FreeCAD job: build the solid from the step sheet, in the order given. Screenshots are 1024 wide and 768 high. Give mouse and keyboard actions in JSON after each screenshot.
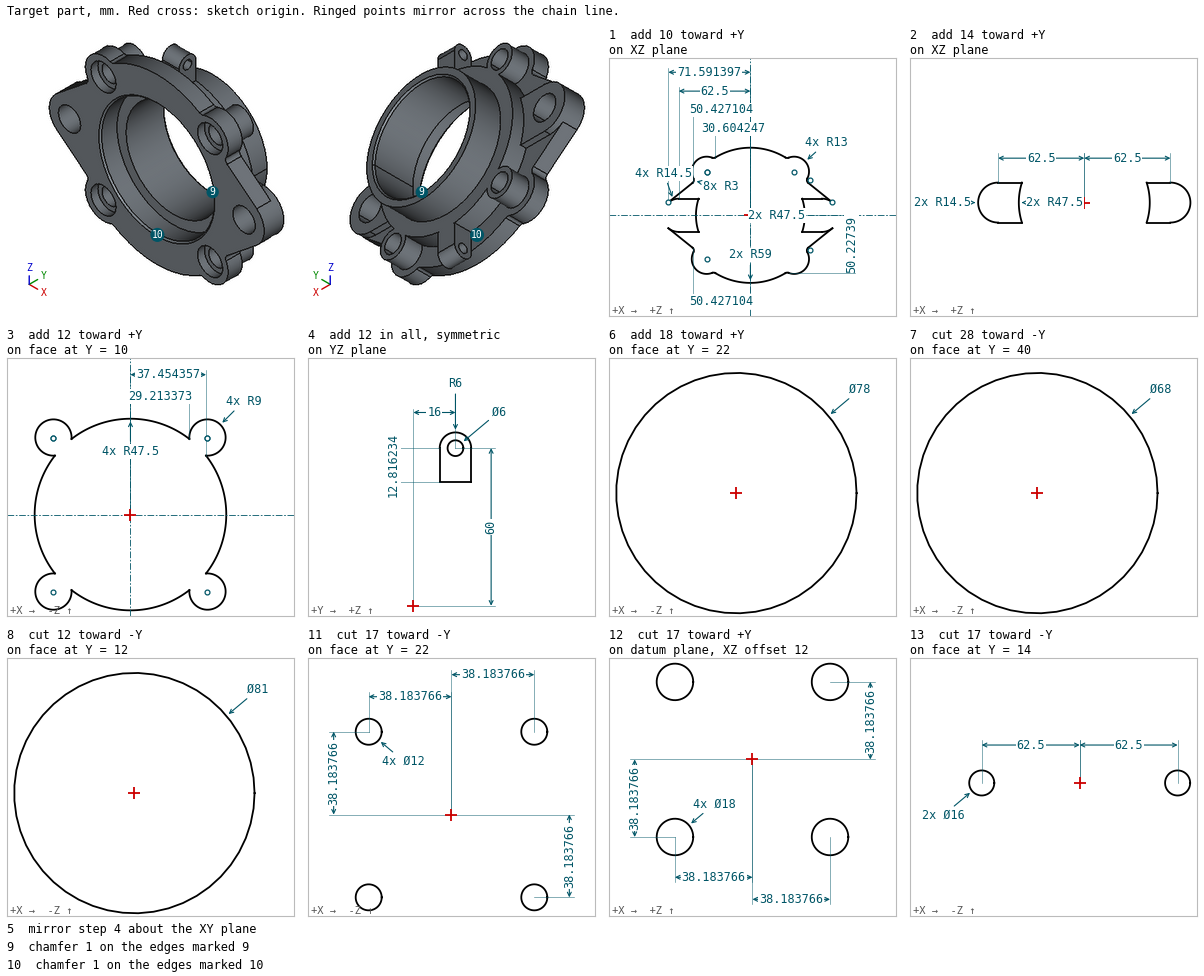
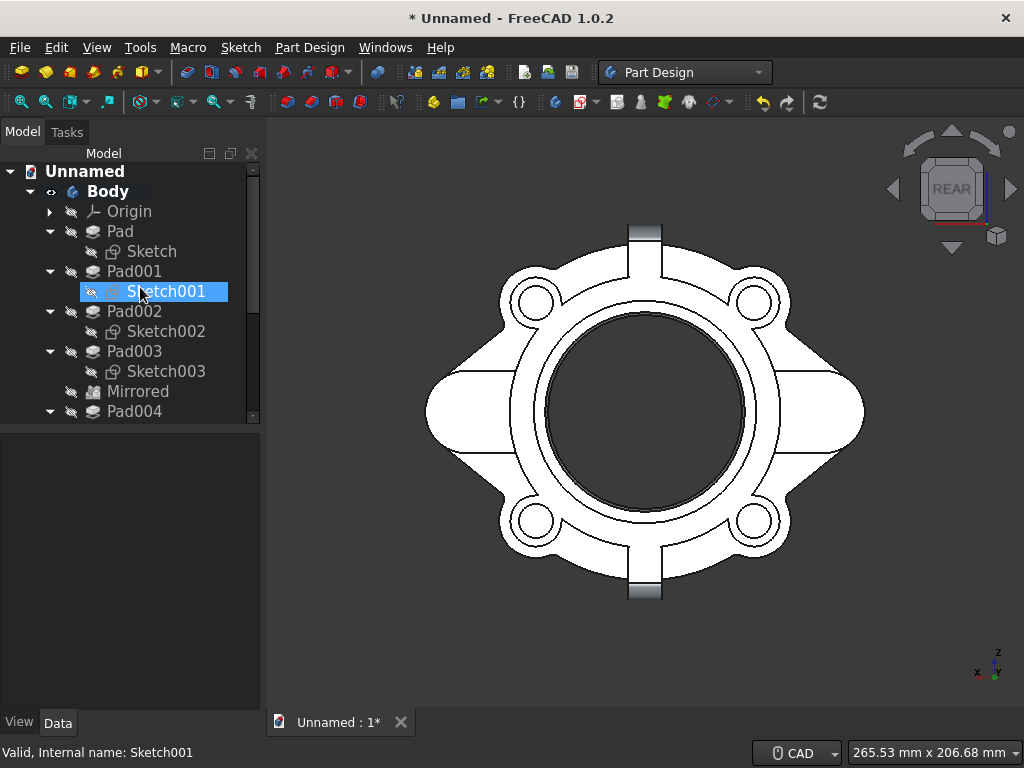
{"action": "left_click", "coordinate": [50, 212]}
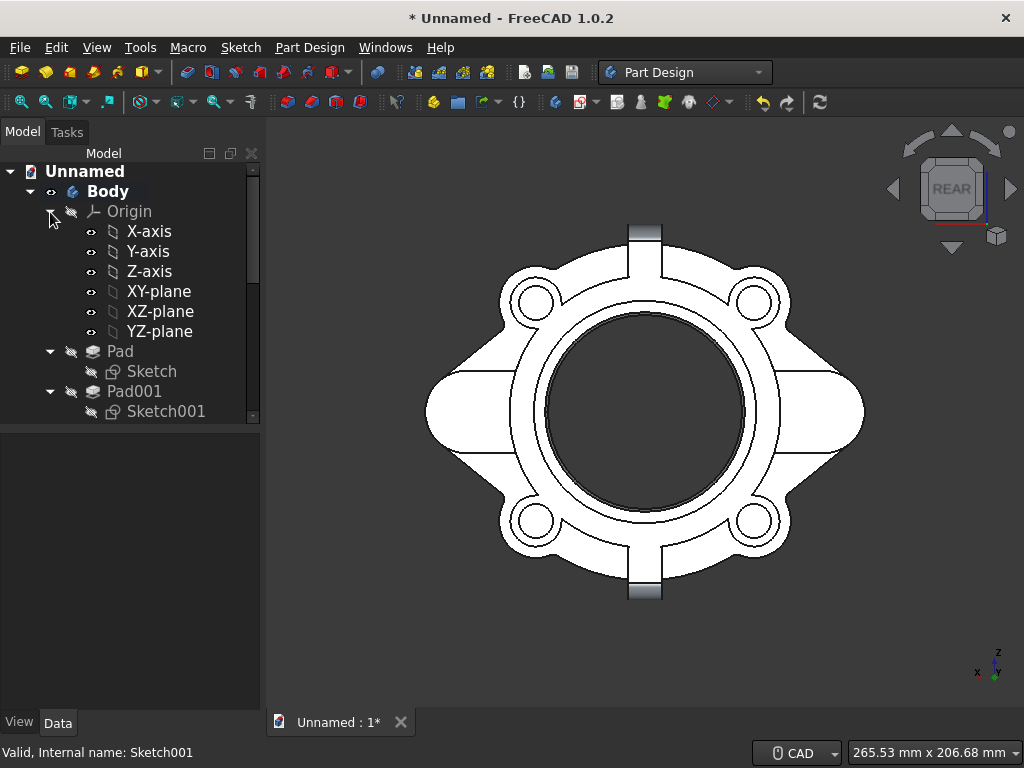
{"action": "left_click", "coordinate": [136, 312]}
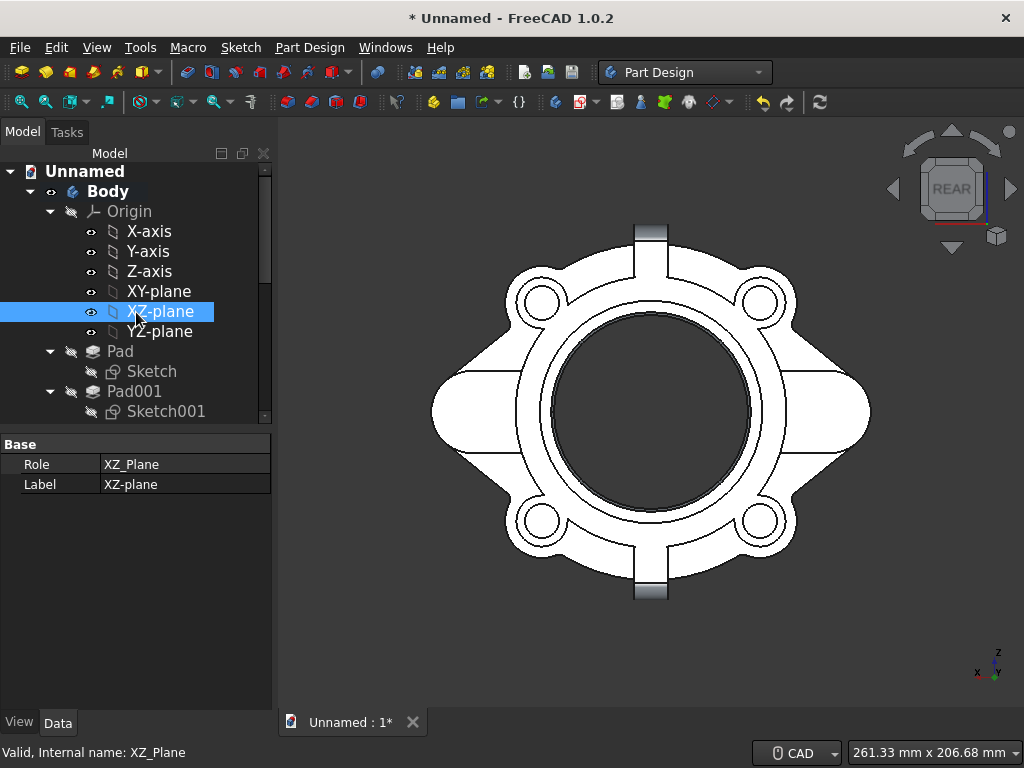
{"action": "left_click", "coordinate": [714, 102]}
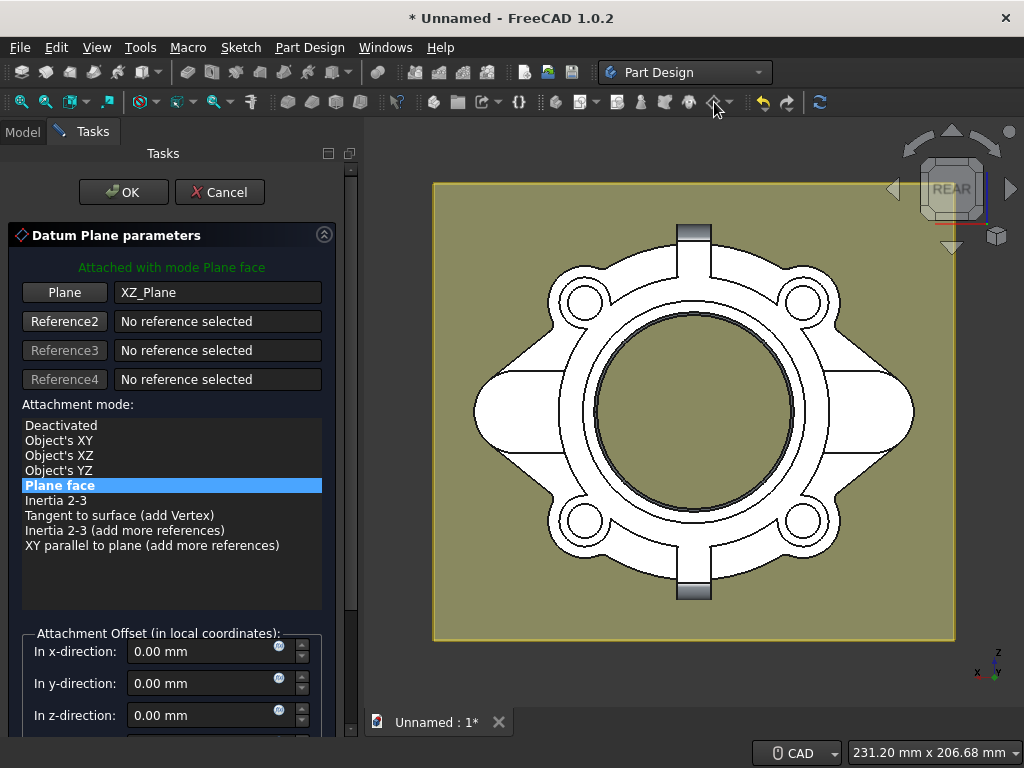
{"action": "triple_click", "coordinate": [210, 715]}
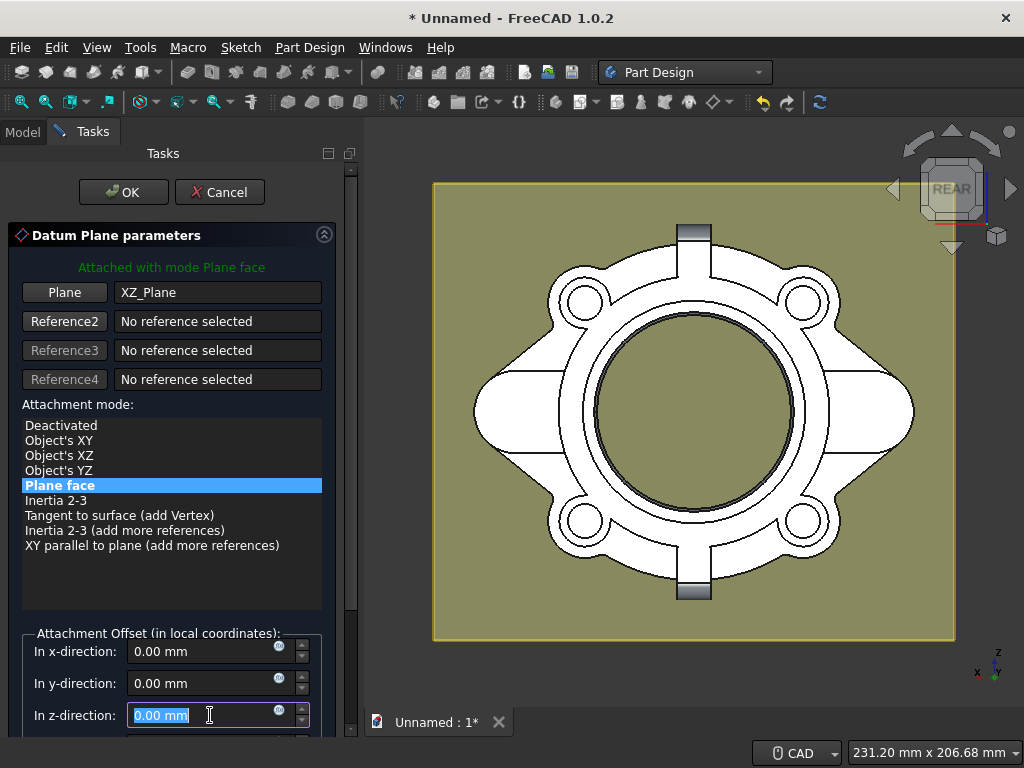
{"action": "type", "text": "12"}
{"action": "key", "text": "Tab"}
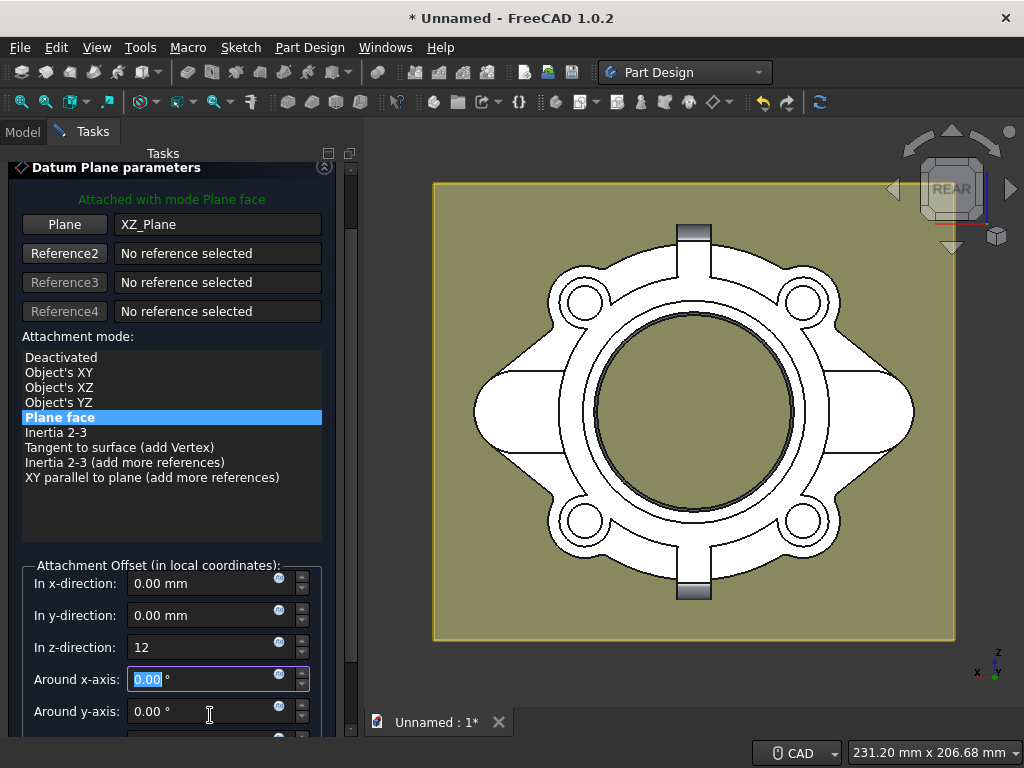
{"action": "scroll", "coordinate": [351, 450], "scroll_direction": "up", "scroll_amount": 2}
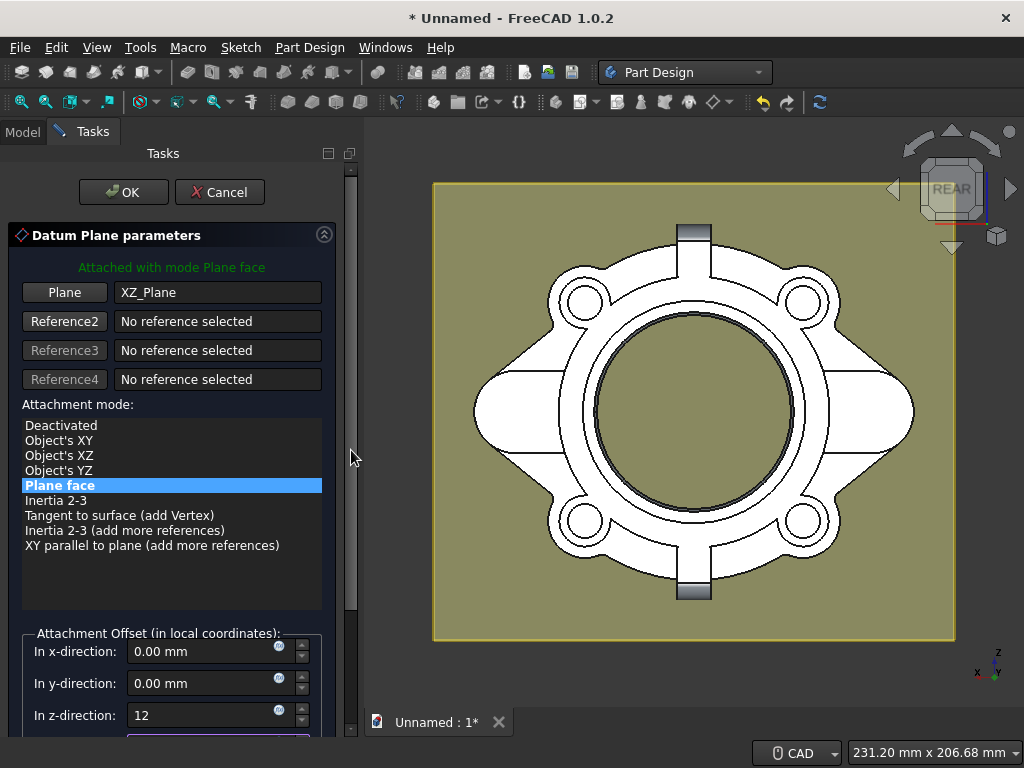
{"action": "left_click", "coordinate": [124, 192]}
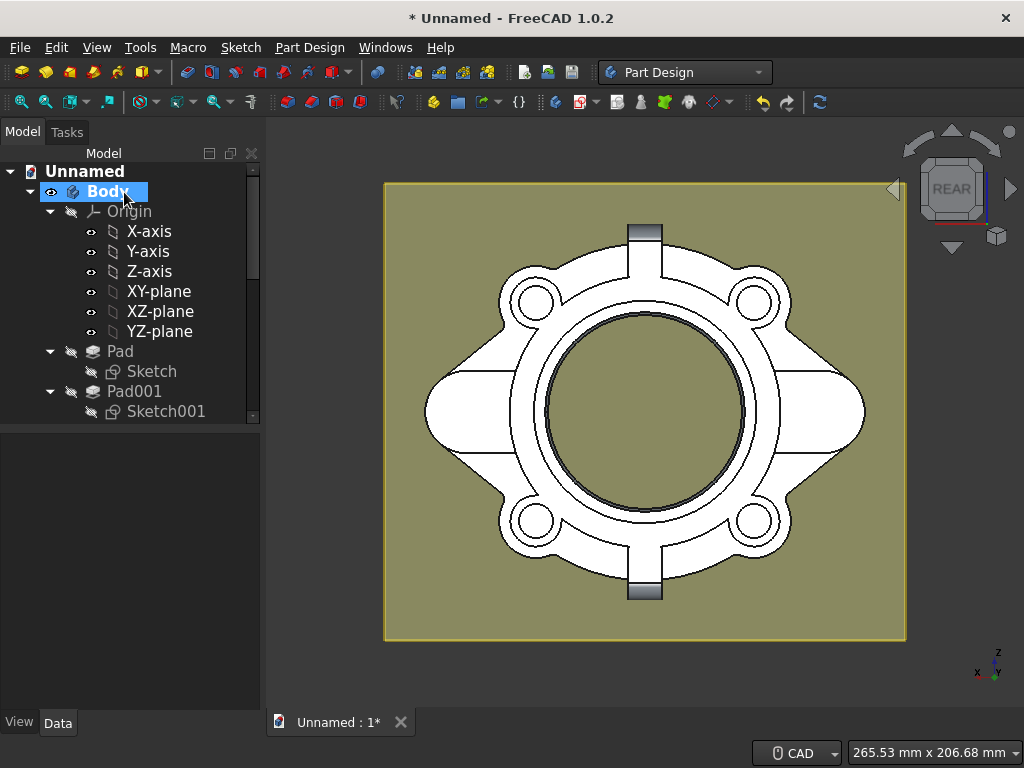
{"action": "scroll", "coordinate": [100, 287], "scroll_direction": "down", "scroll_amount": 3}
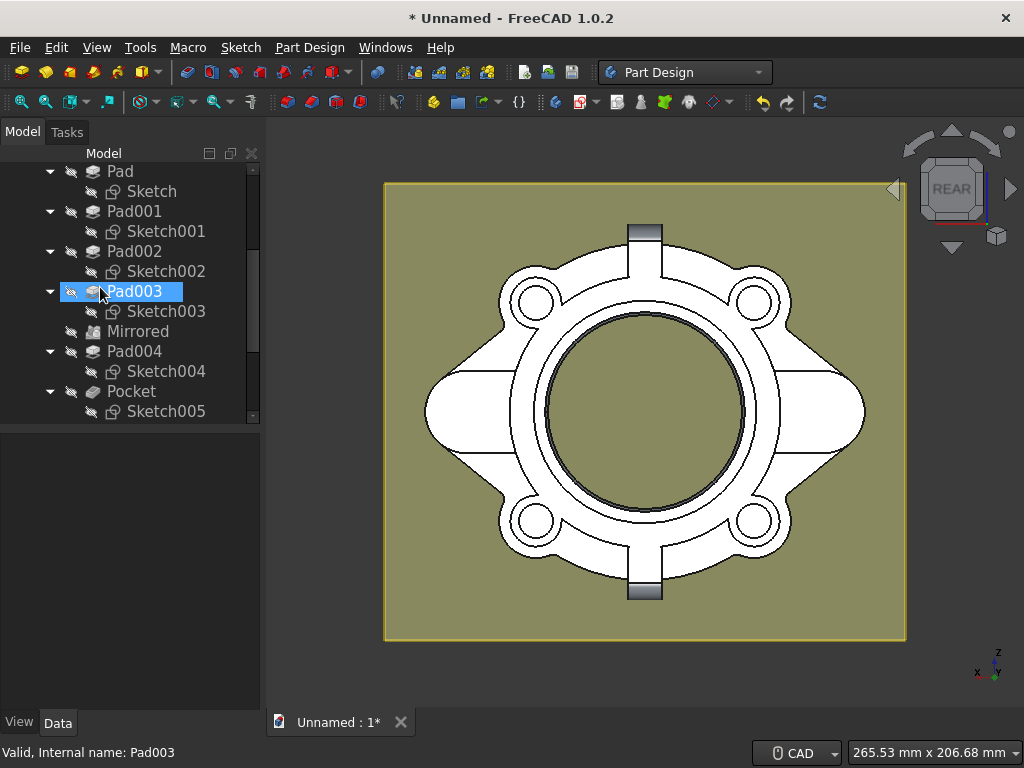
{"action": "scroll", "coordinate": [140, 287], "scroll_direction": "up", "scroll_amount": 15}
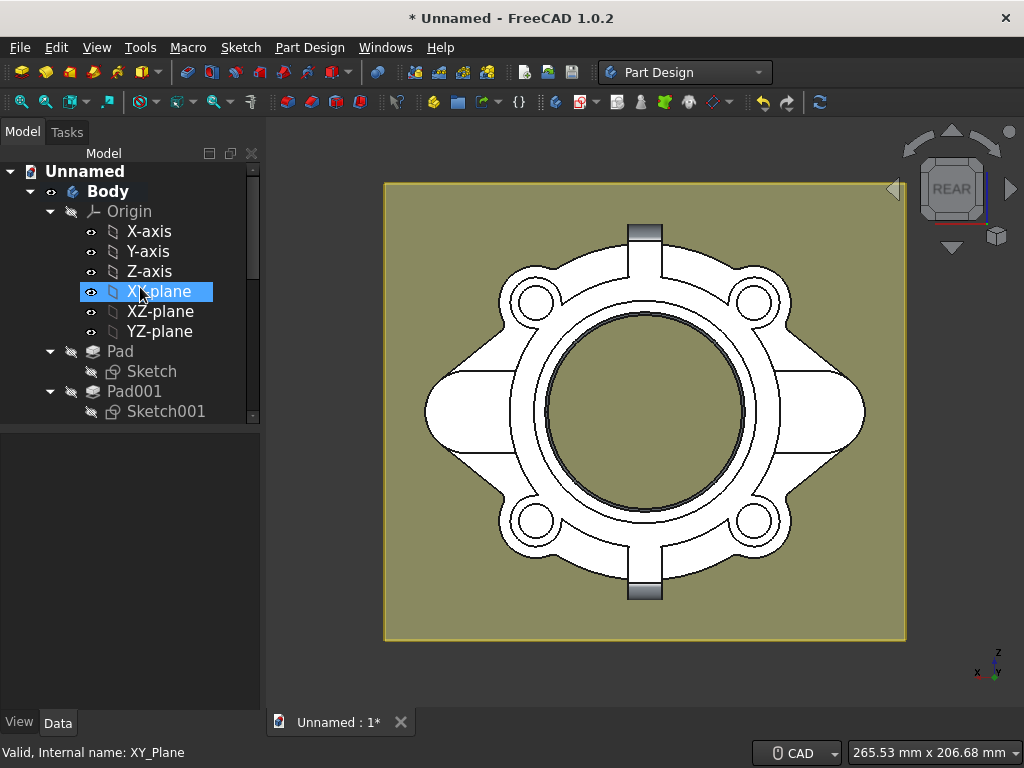
{"action": "scroll", "coordinate": [100, 287], "scroll_direction": "down", "scroll_amount": 6}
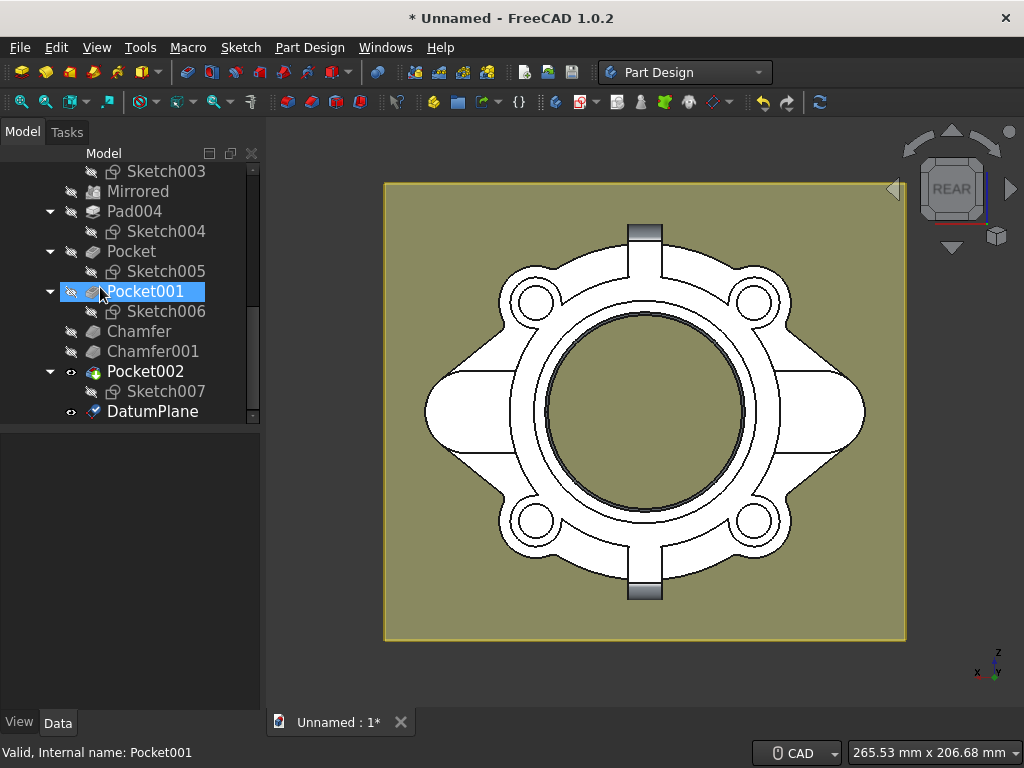
{"action": "left_click", "coordinate": [116, 412]}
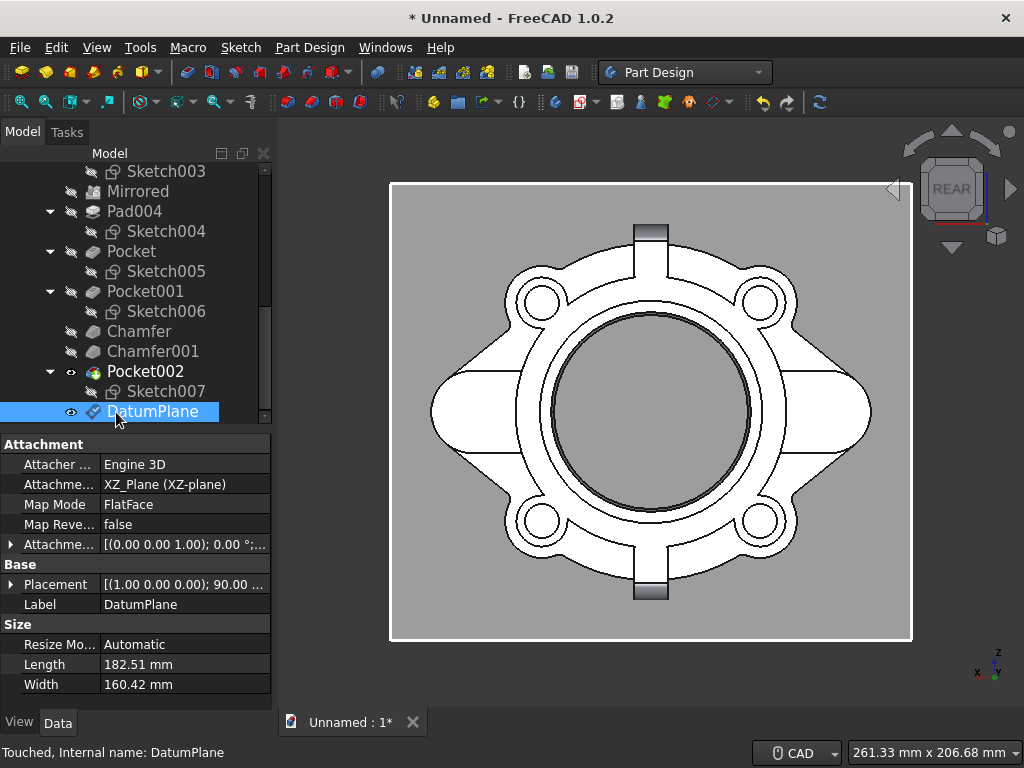
{"action": "left_click", "coordinate": [580, 102]}